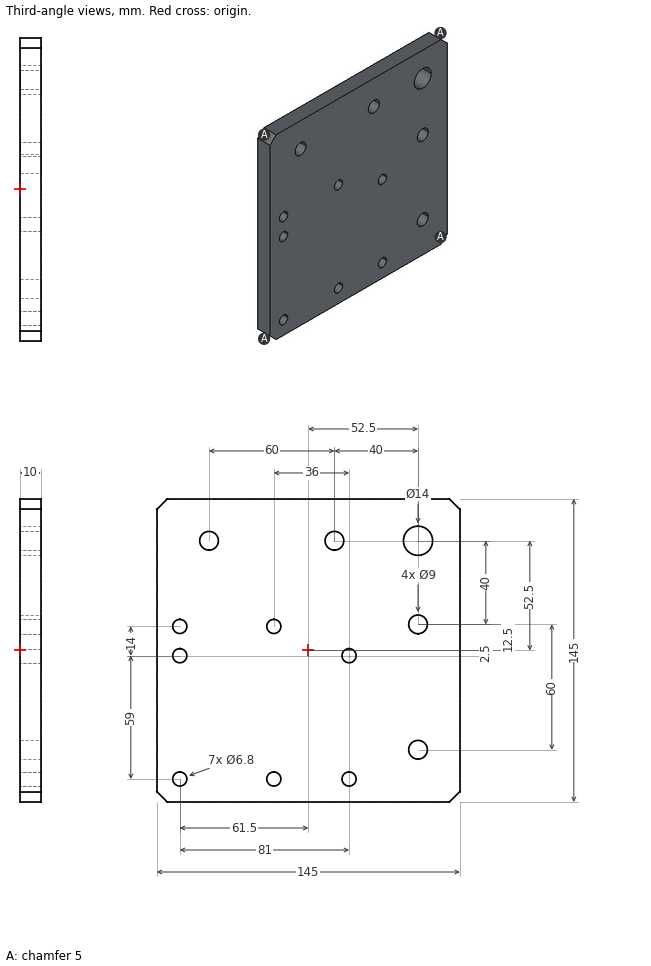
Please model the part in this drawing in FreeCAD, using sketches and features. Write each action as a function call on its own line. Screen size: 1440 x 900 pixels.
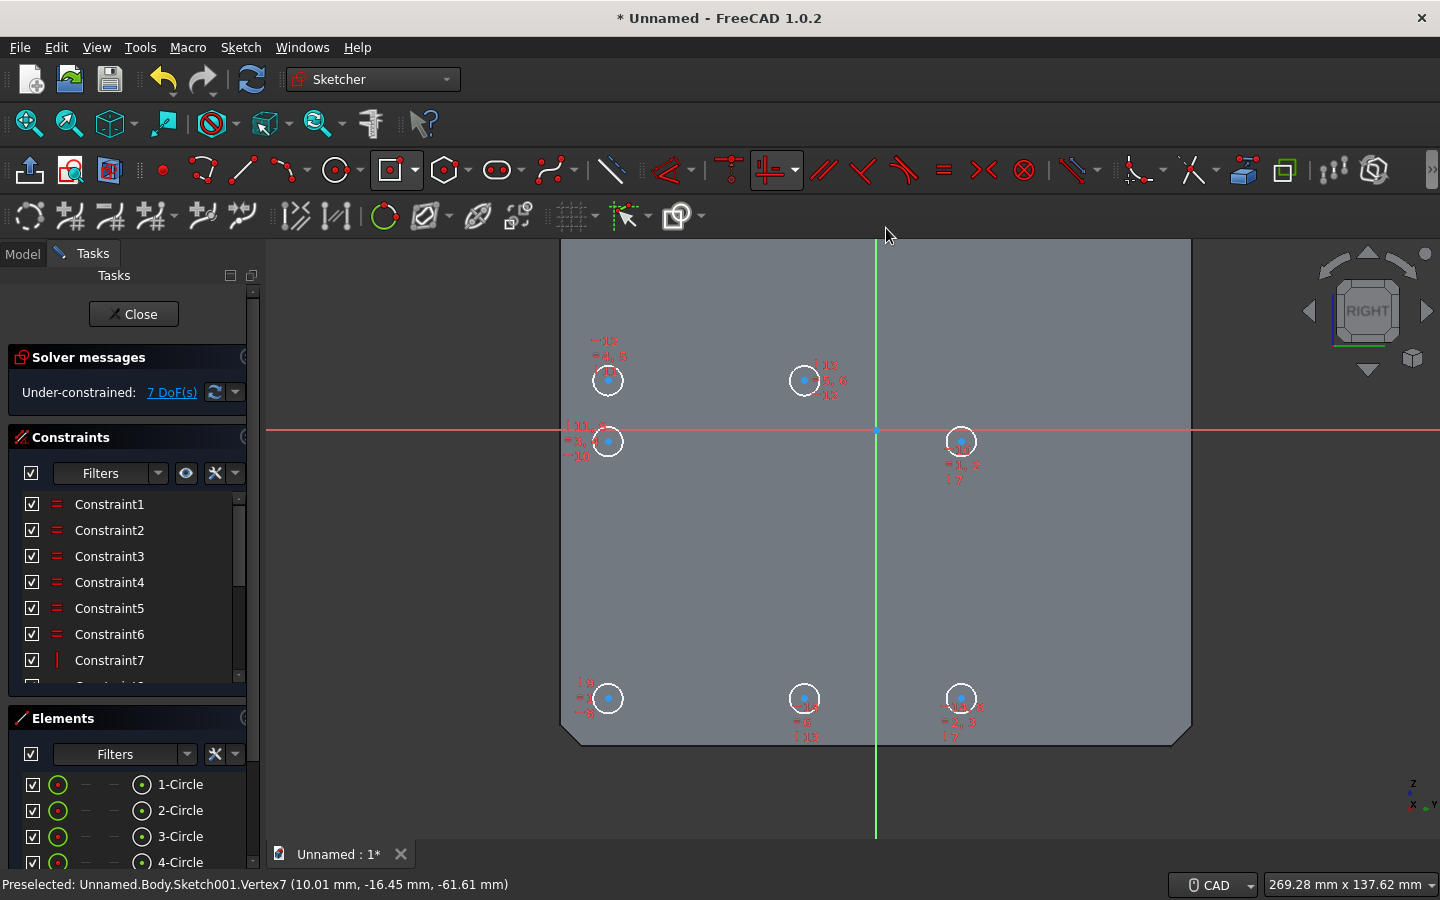
scroll(618, 688, up, 2)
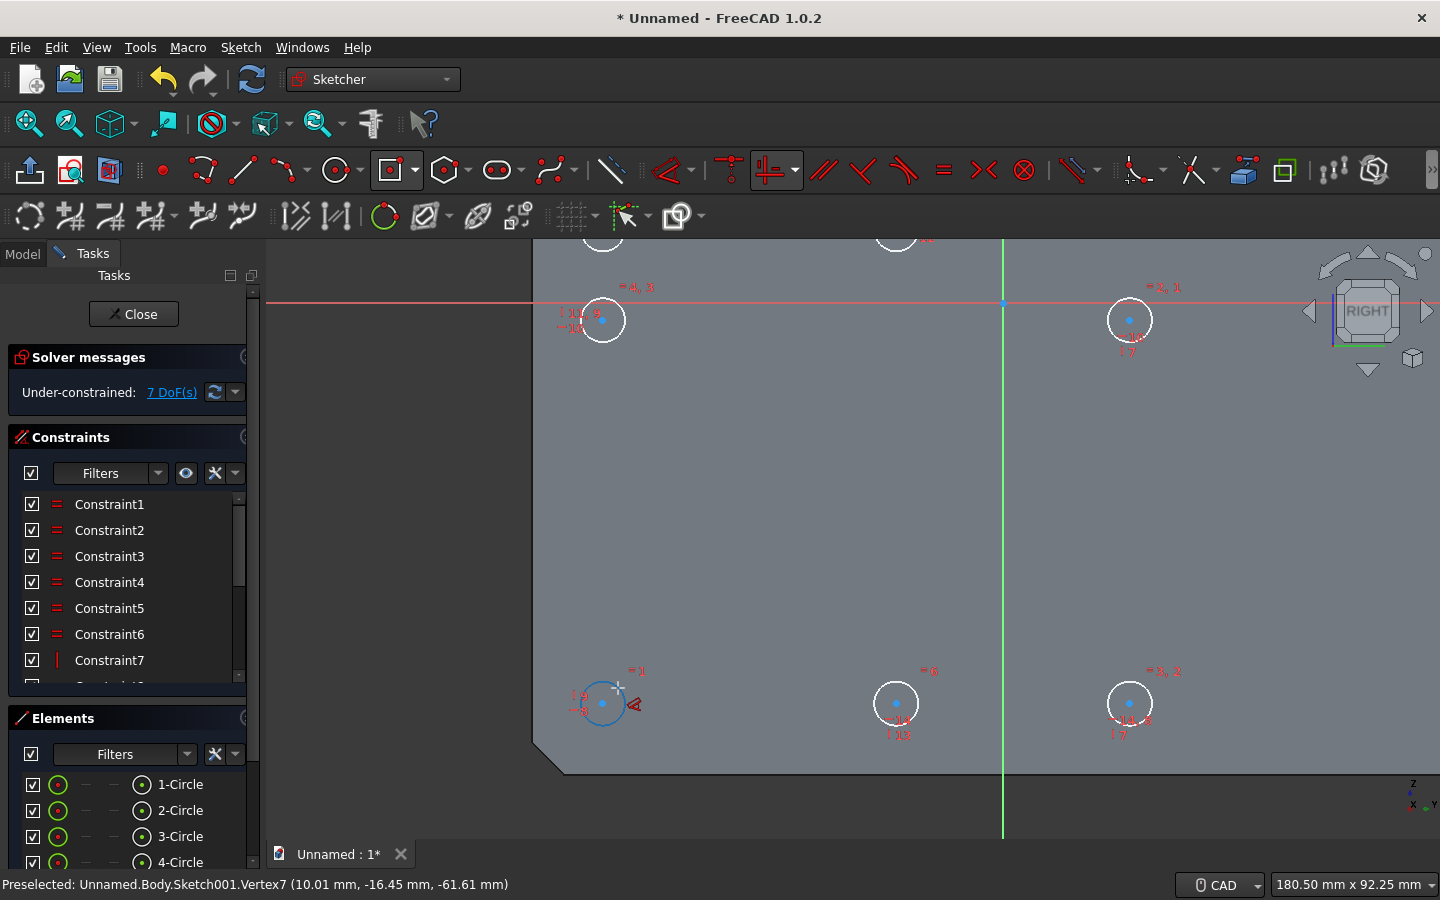
click(618, 688)
click(640, 665)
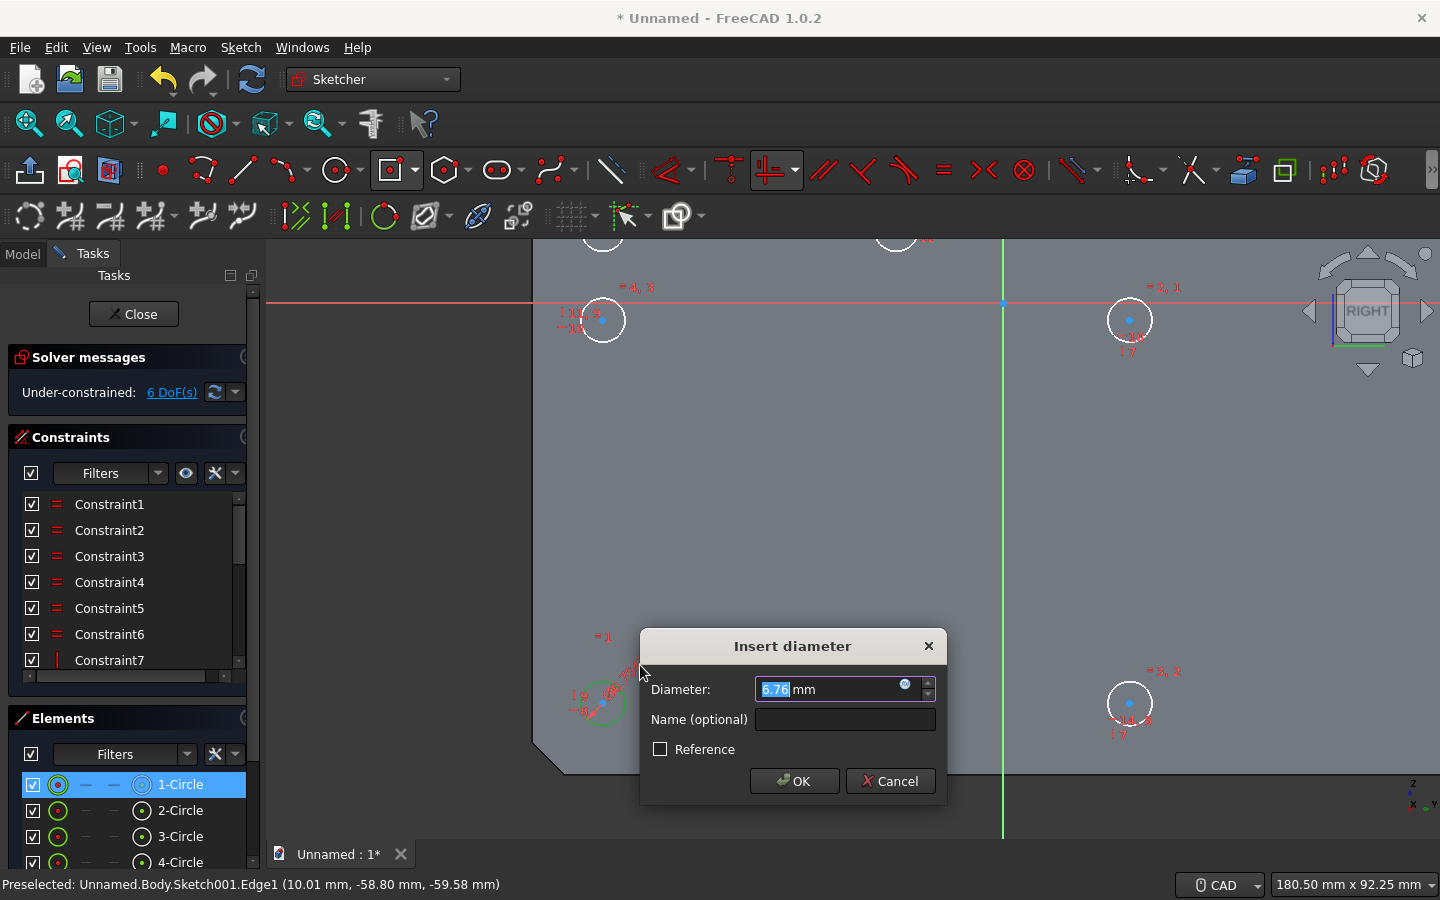
text(6.8)
key(Return)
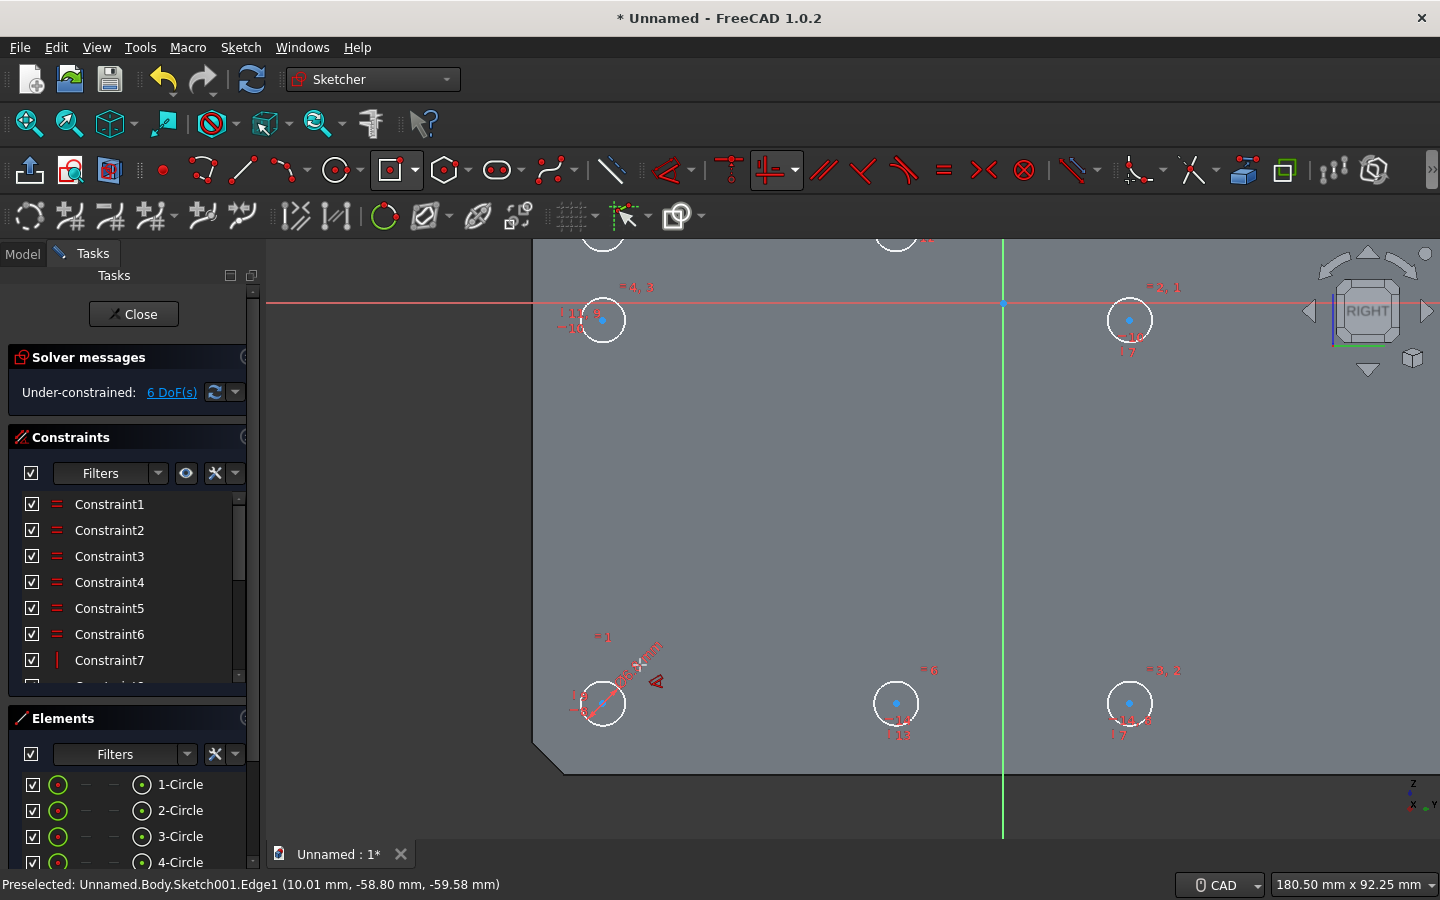
scroll(1130, 320, up, 5)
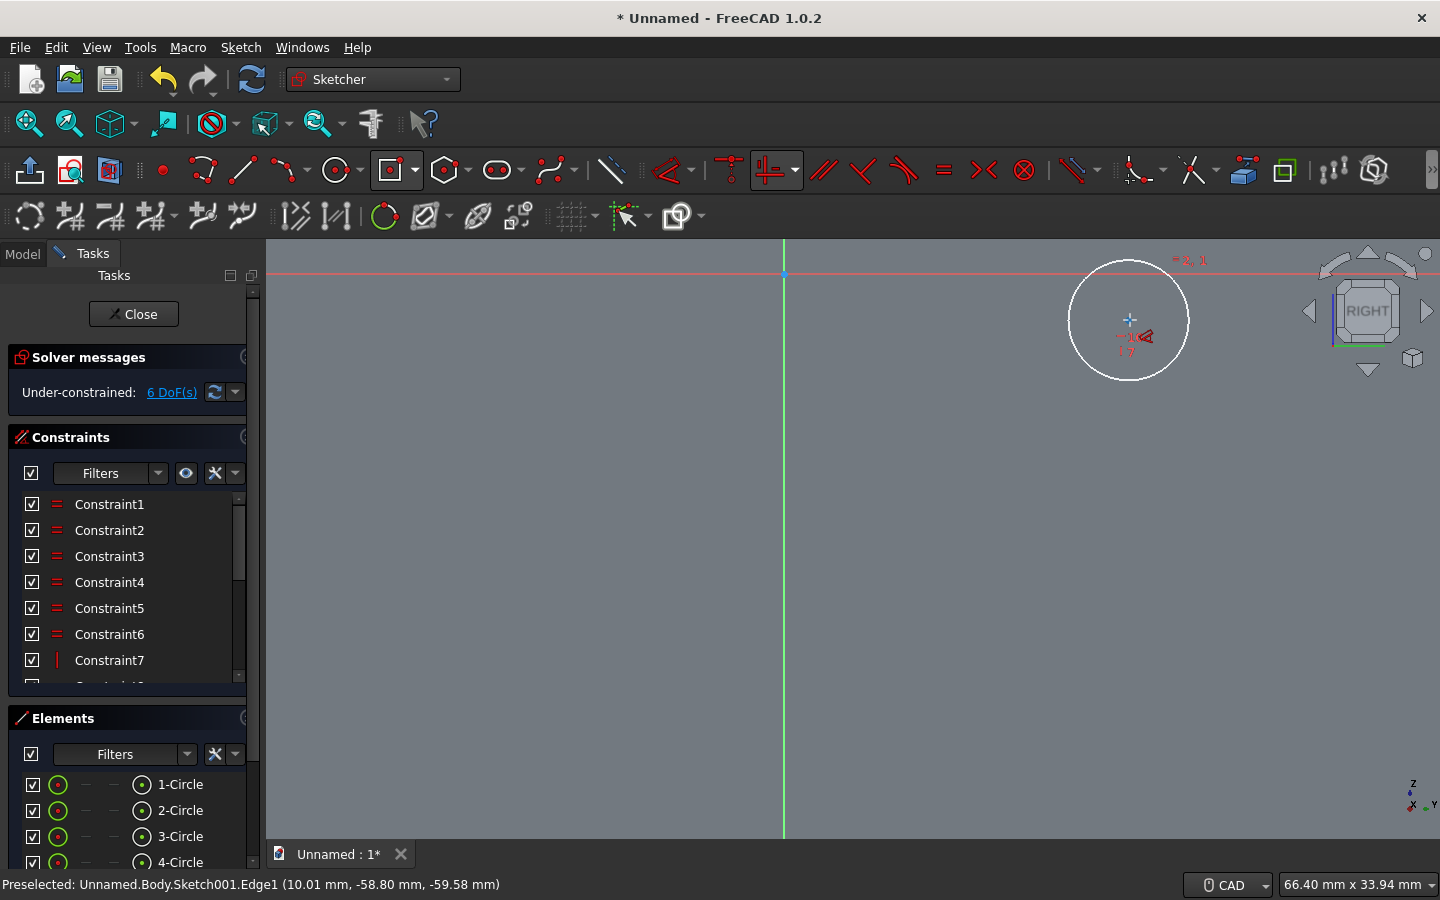
click(1129, 320)
click(1163, 297)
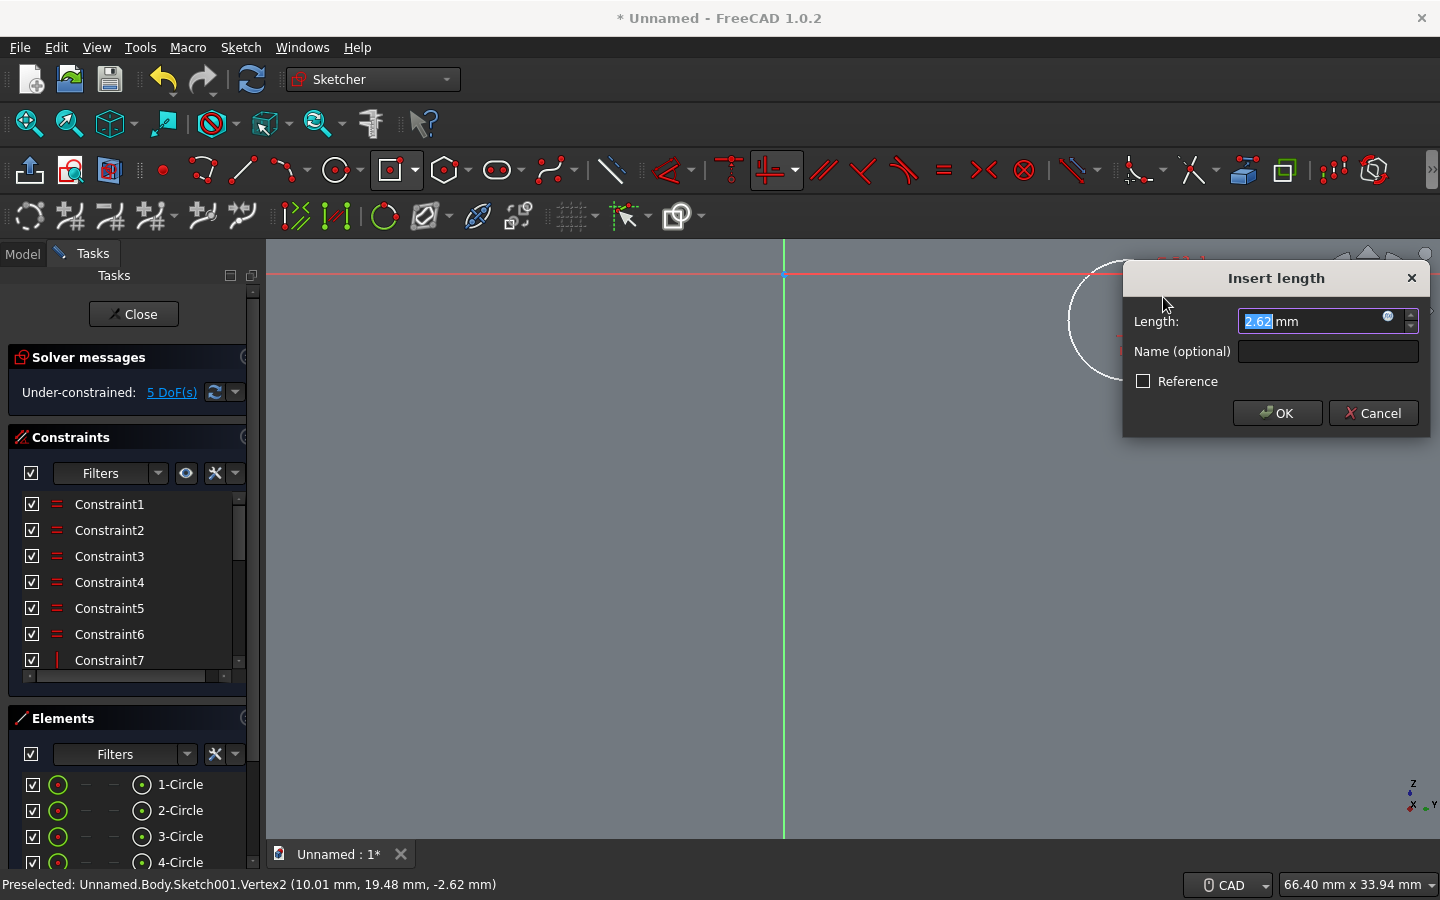
text(2.5)
key(Return)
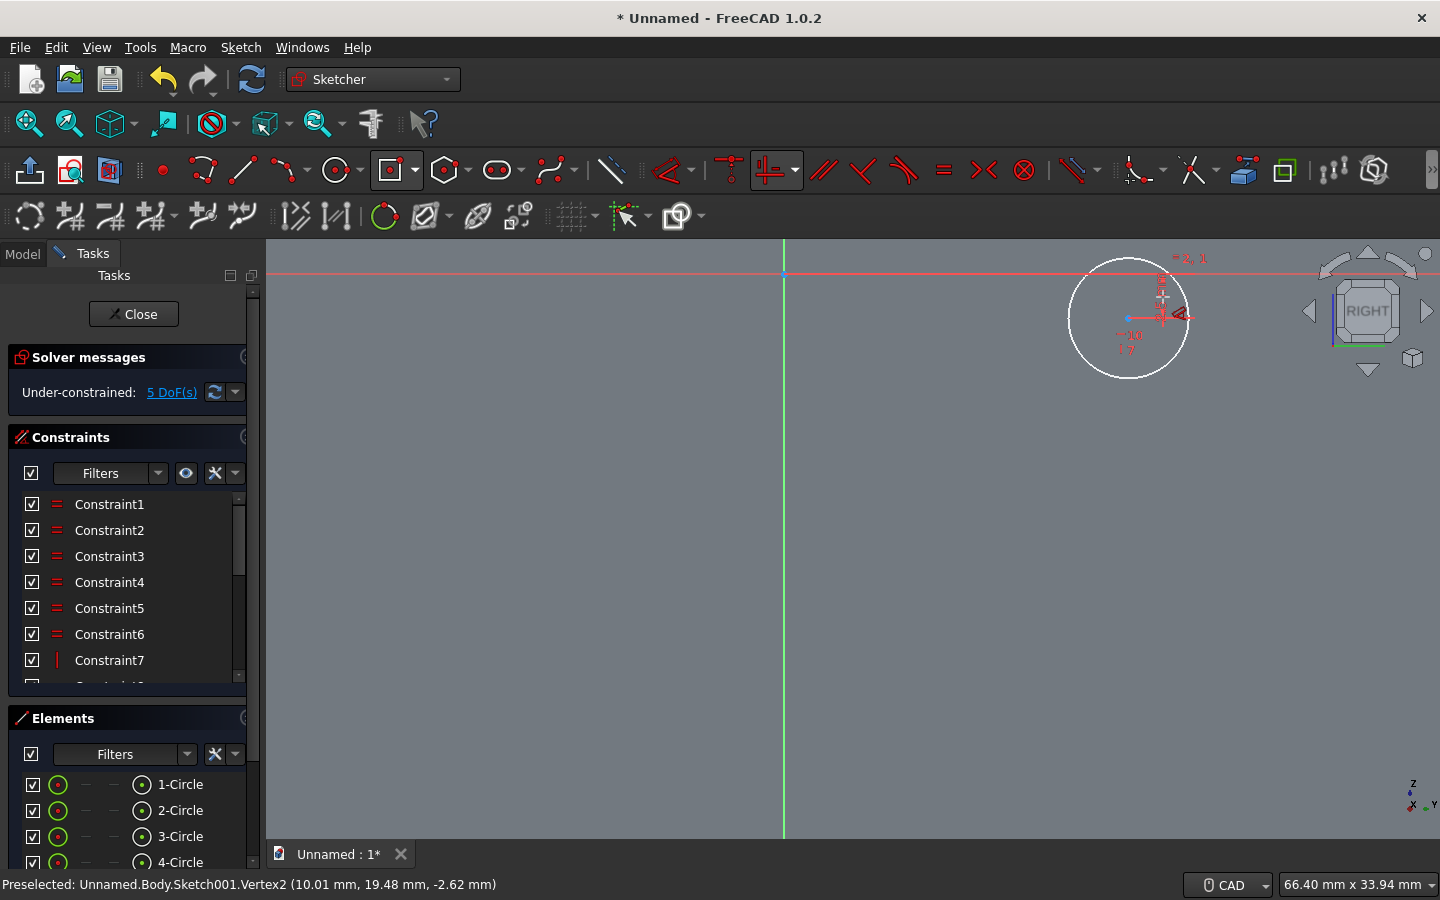
scroll(906, 481, down, 7)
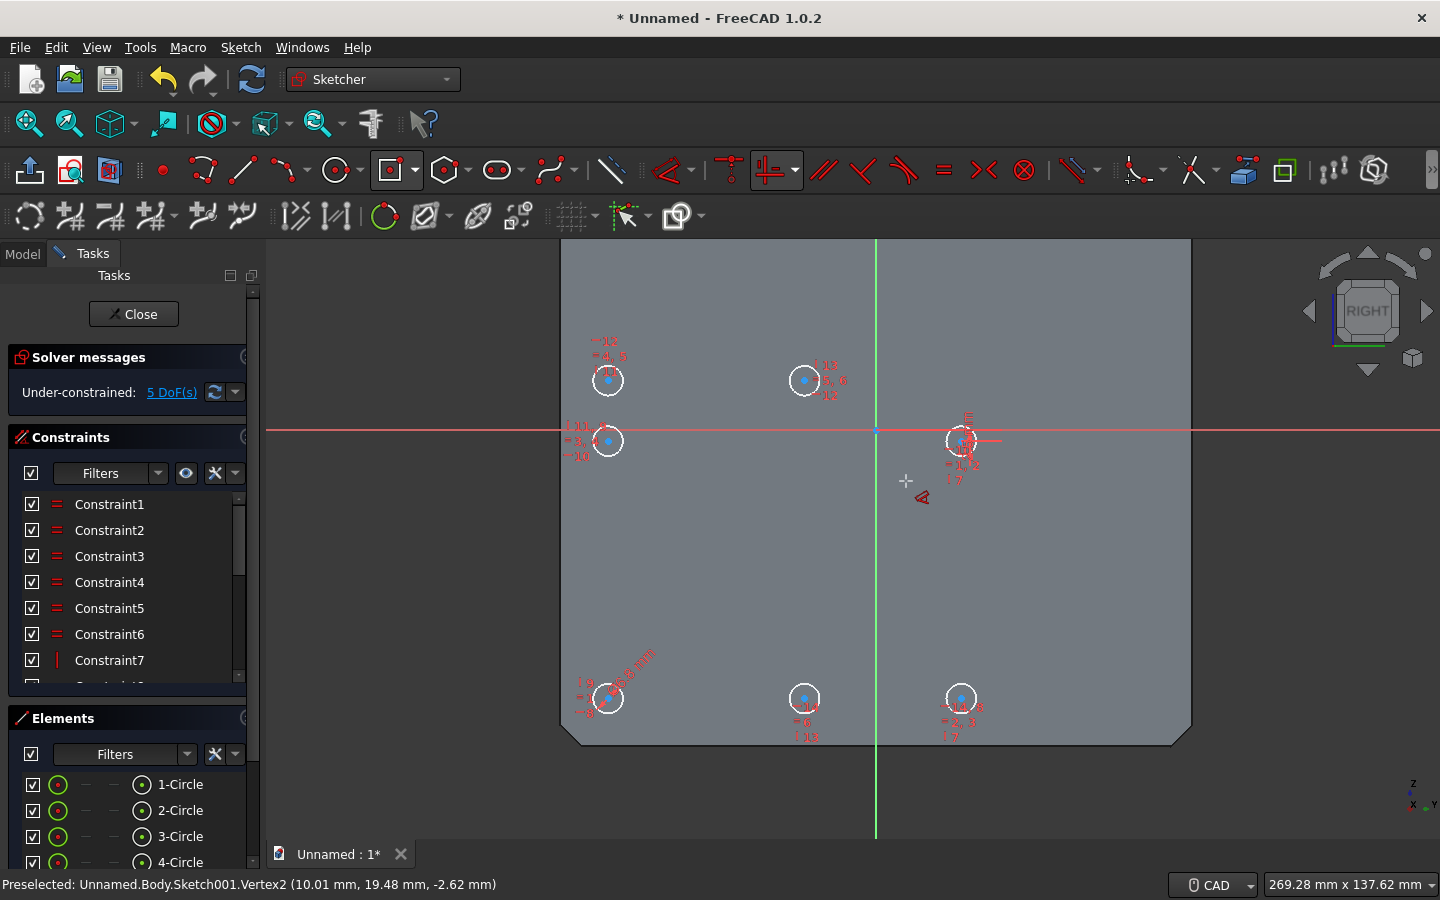
click(608, 699)